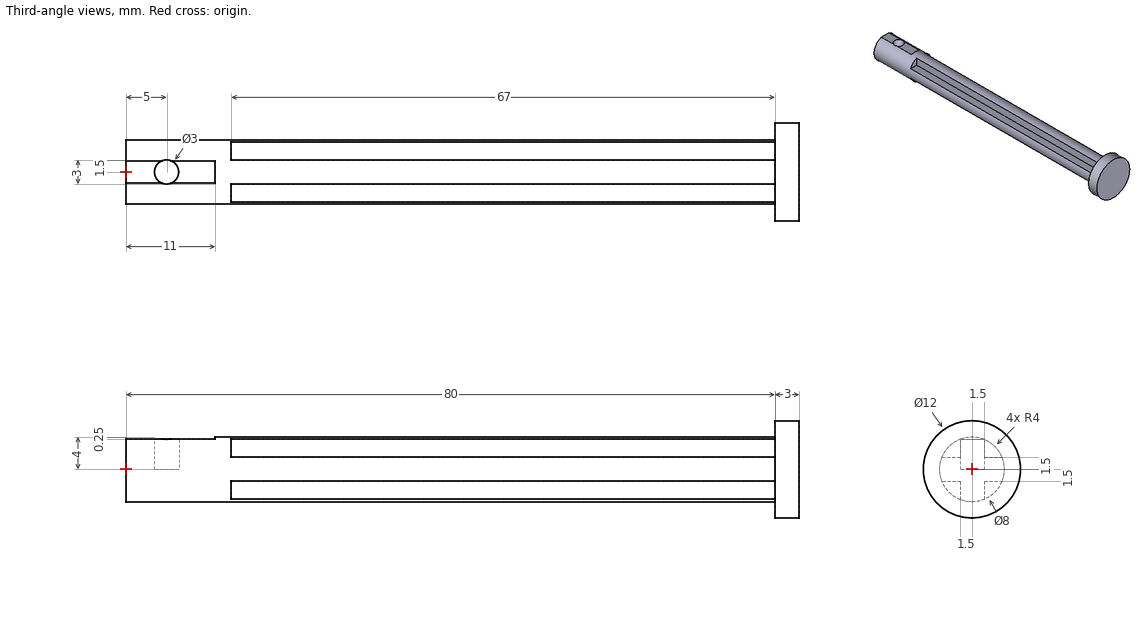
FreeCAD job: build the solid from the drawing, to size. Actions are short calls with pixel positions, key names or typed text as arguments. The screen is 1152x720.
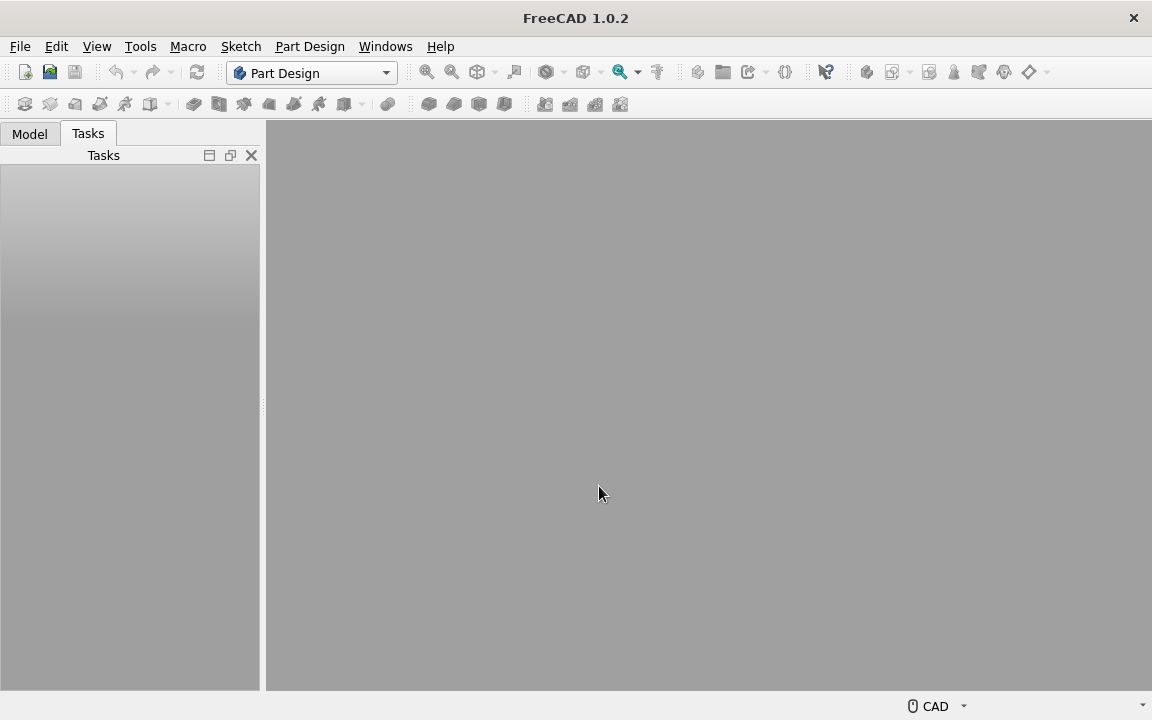
key(ctrl+n)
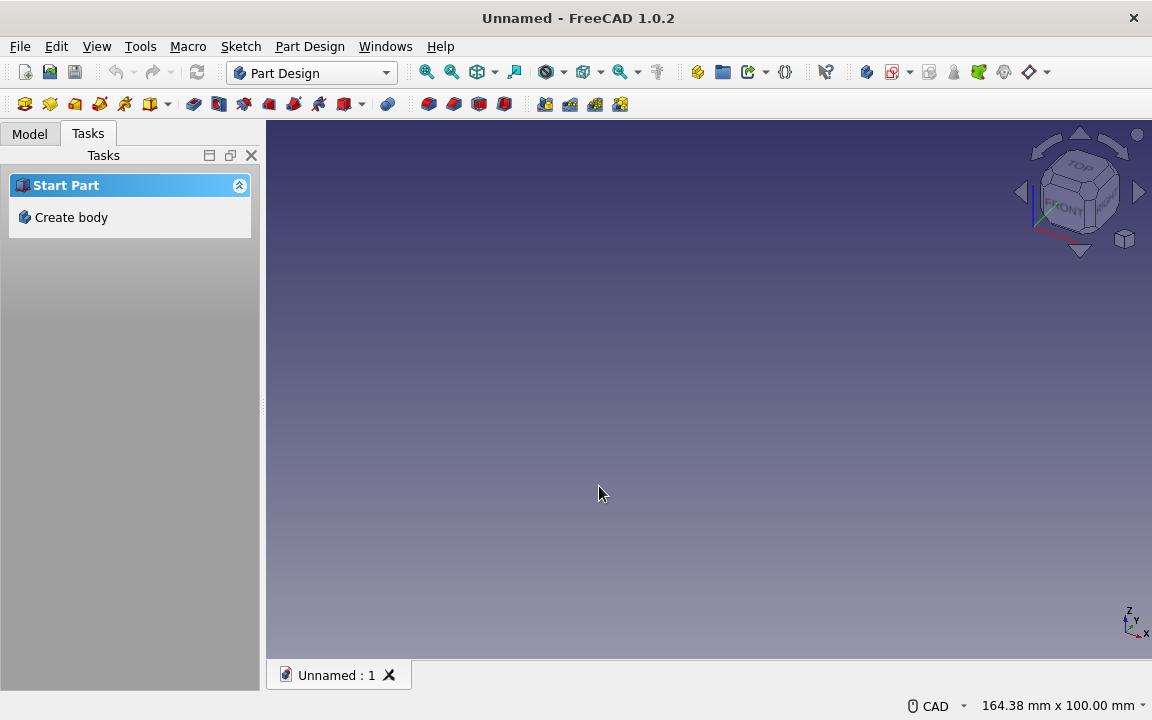
click(892, 72)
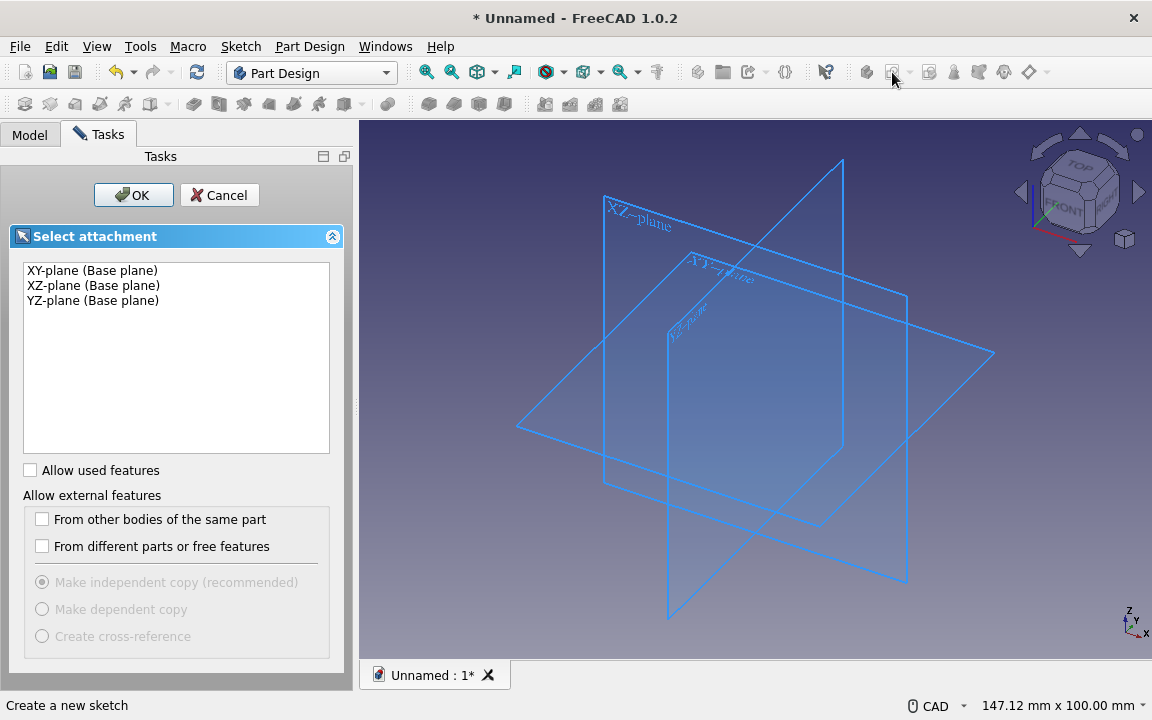
click(84, 300)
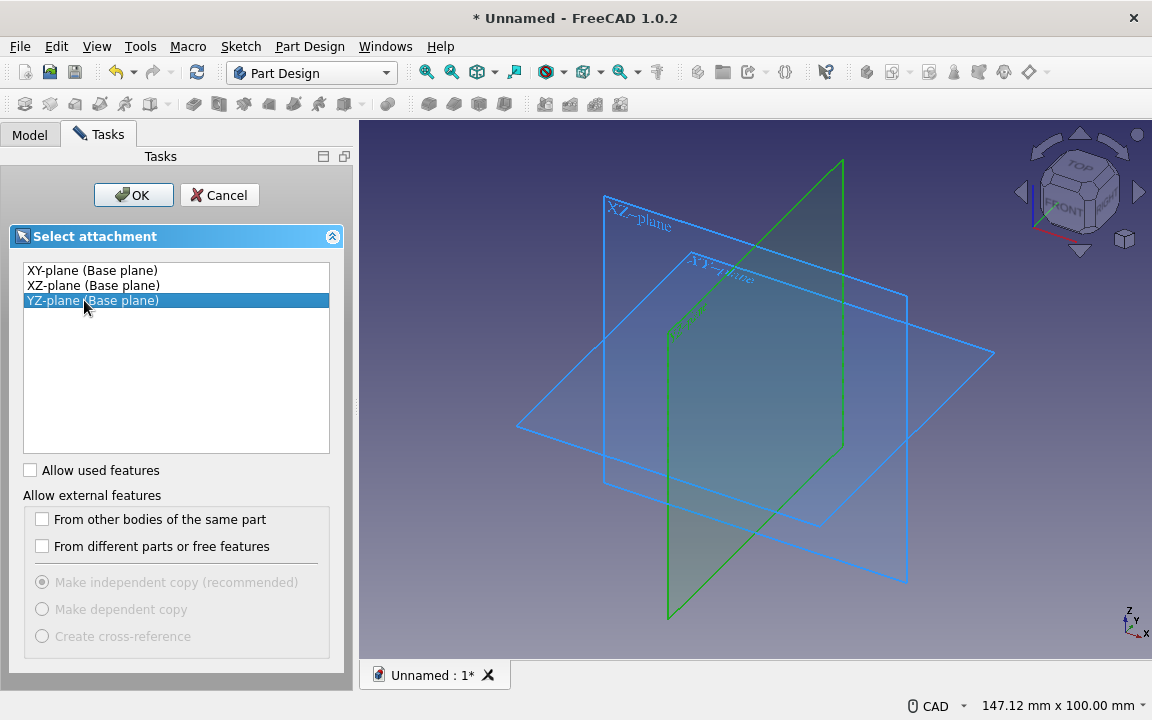
click(134, 195)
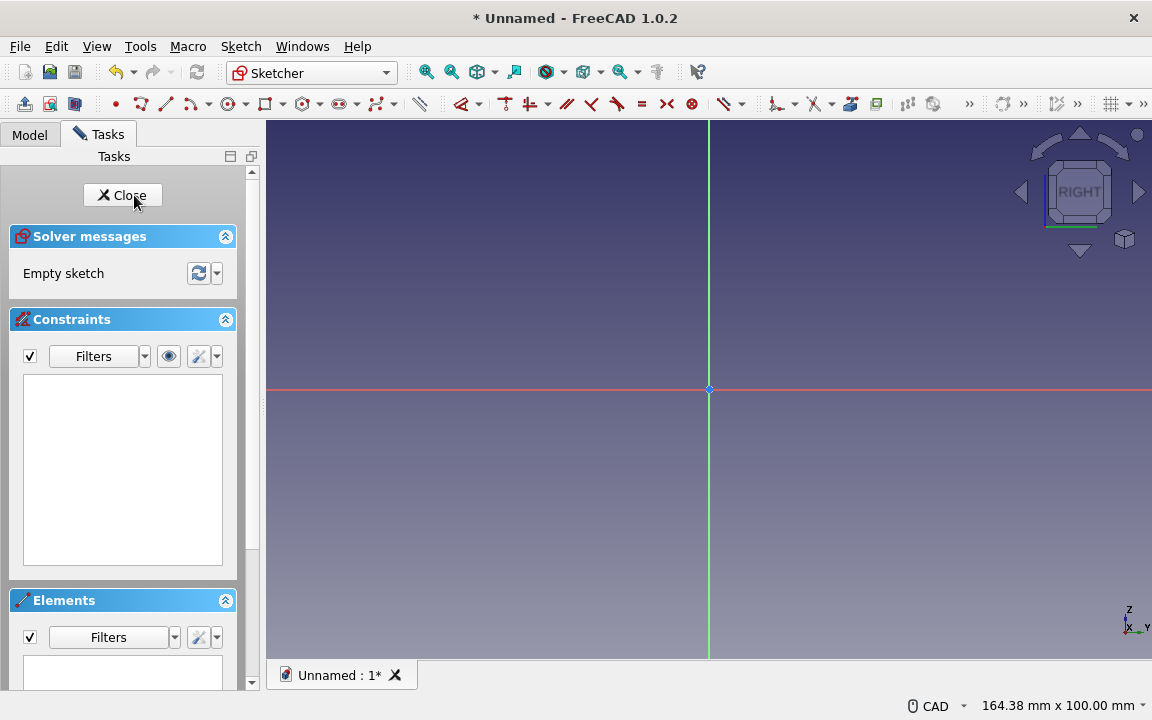
scroll(720, 390, up, 10)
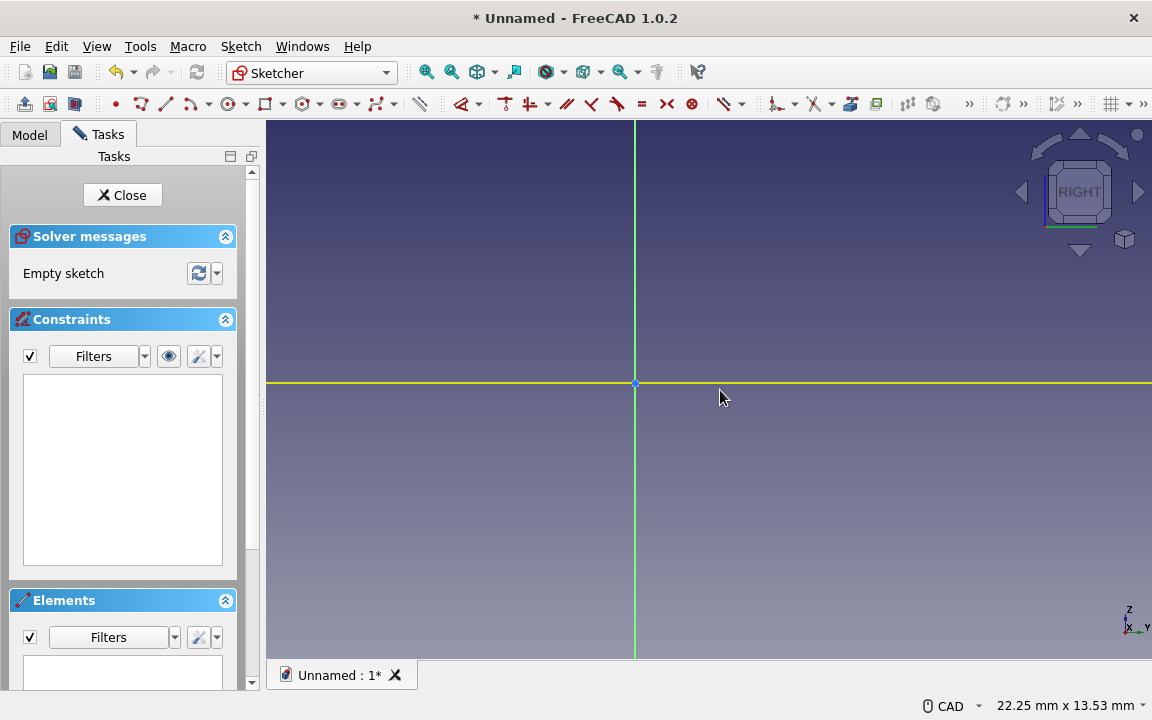
click(228, 104)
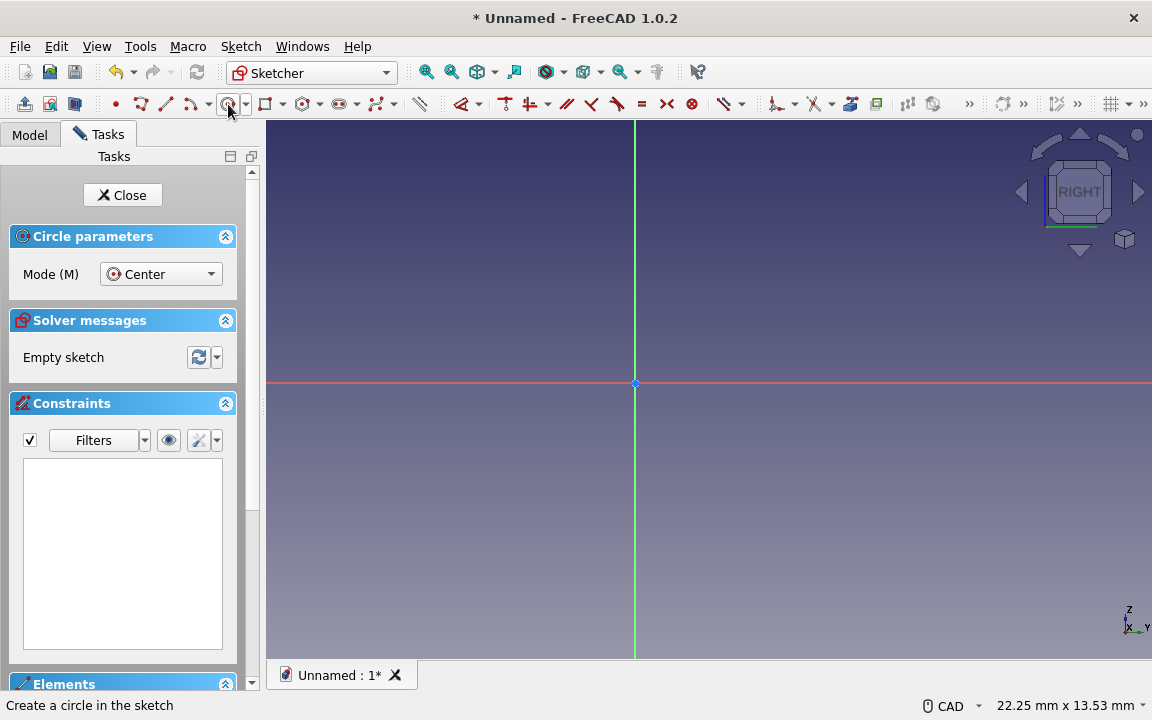
click(635, 383)
move(748, 270)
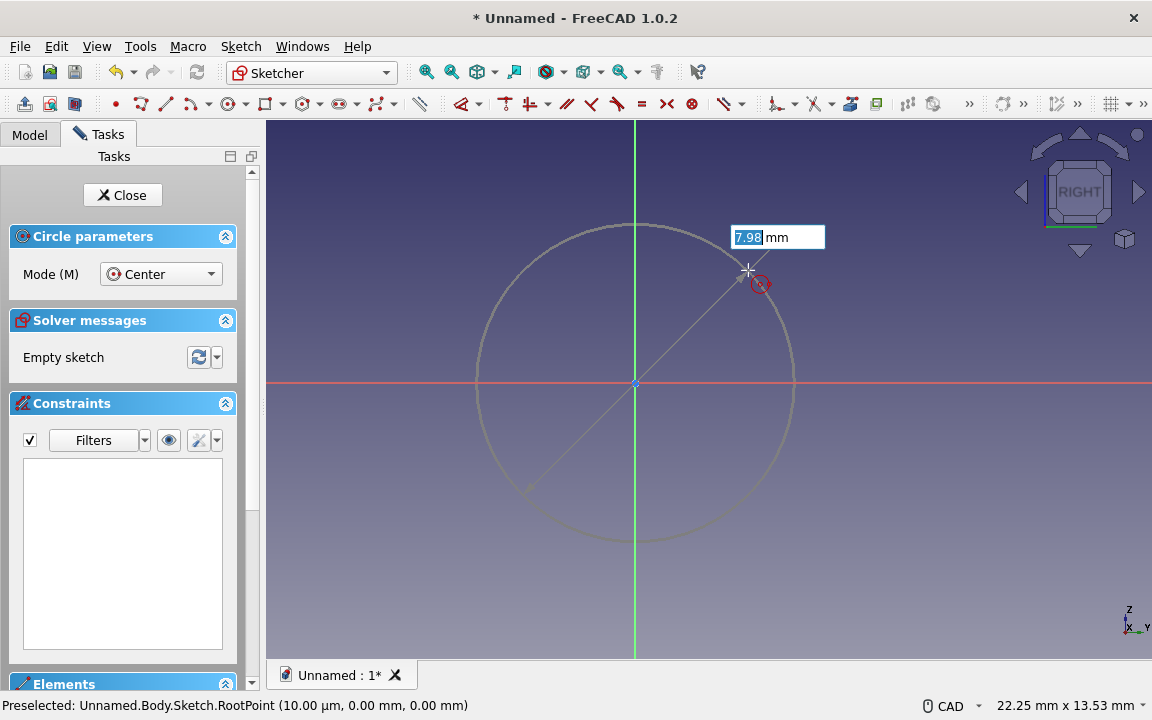
text(8)
key(Return)
key(Escape)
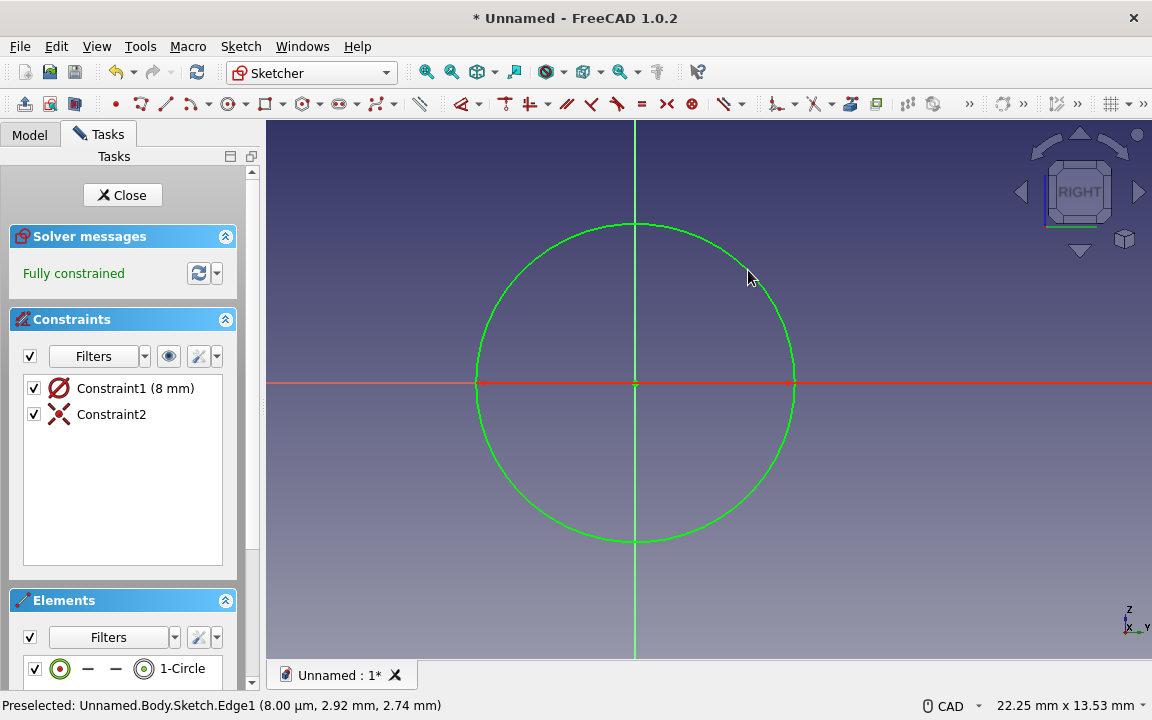
click(123, 195)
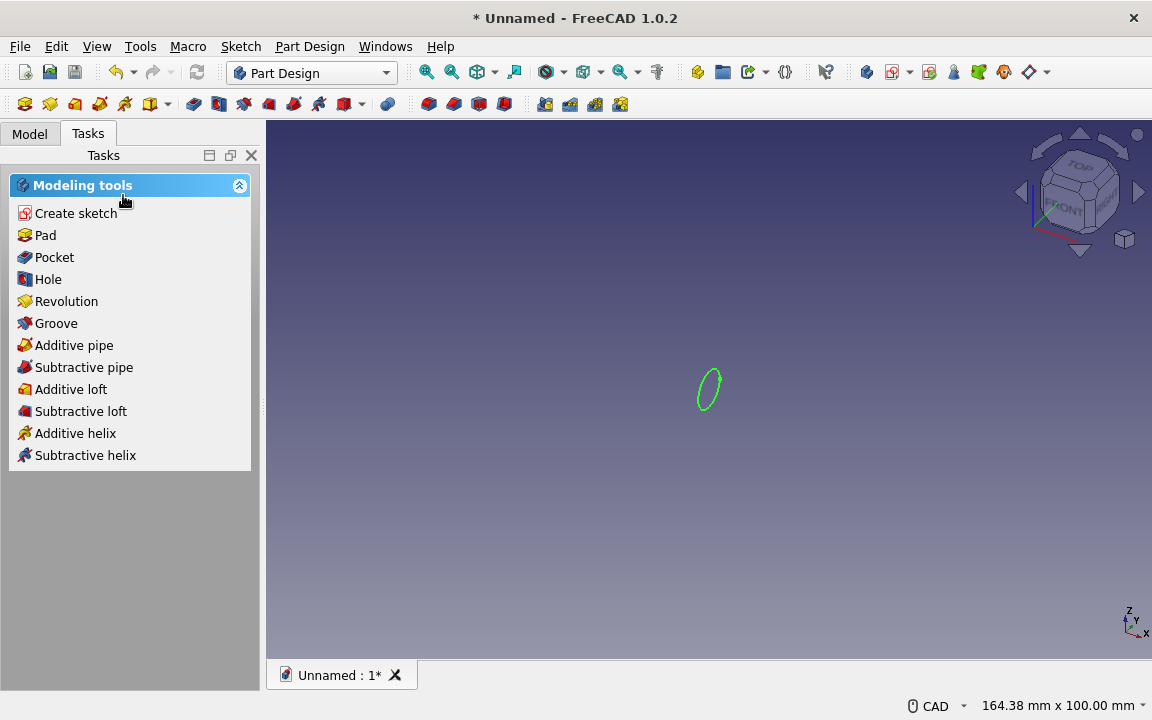
click(25, 104)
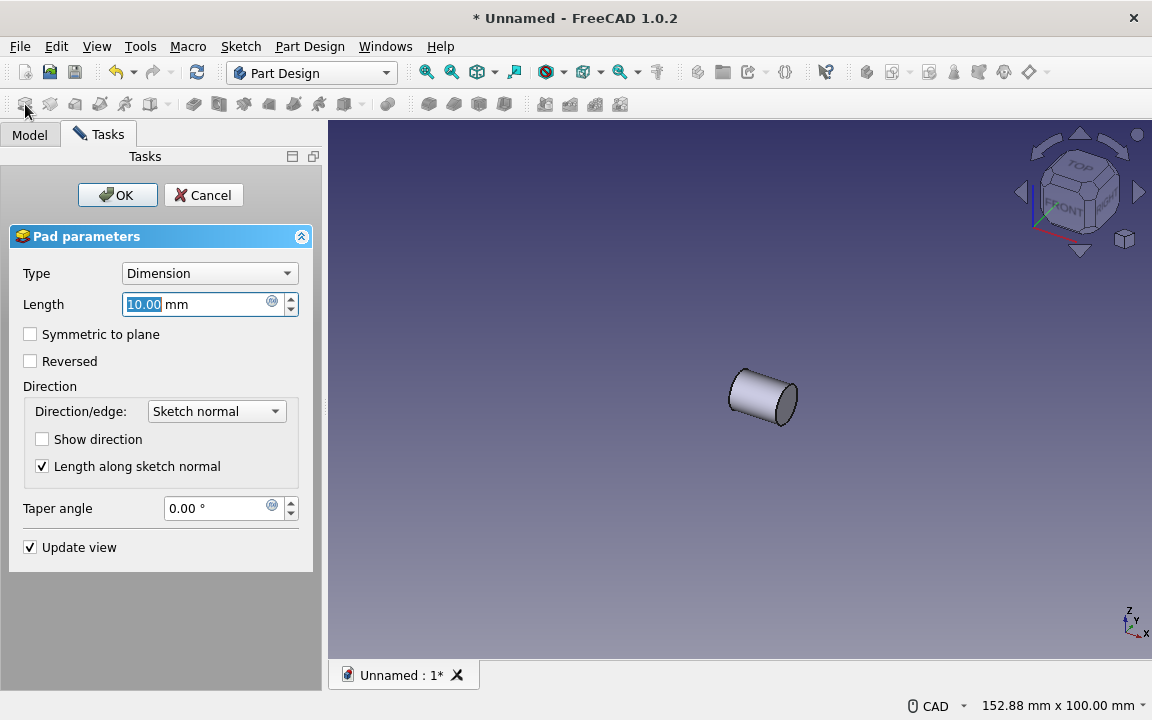
text(80)
key(Tab)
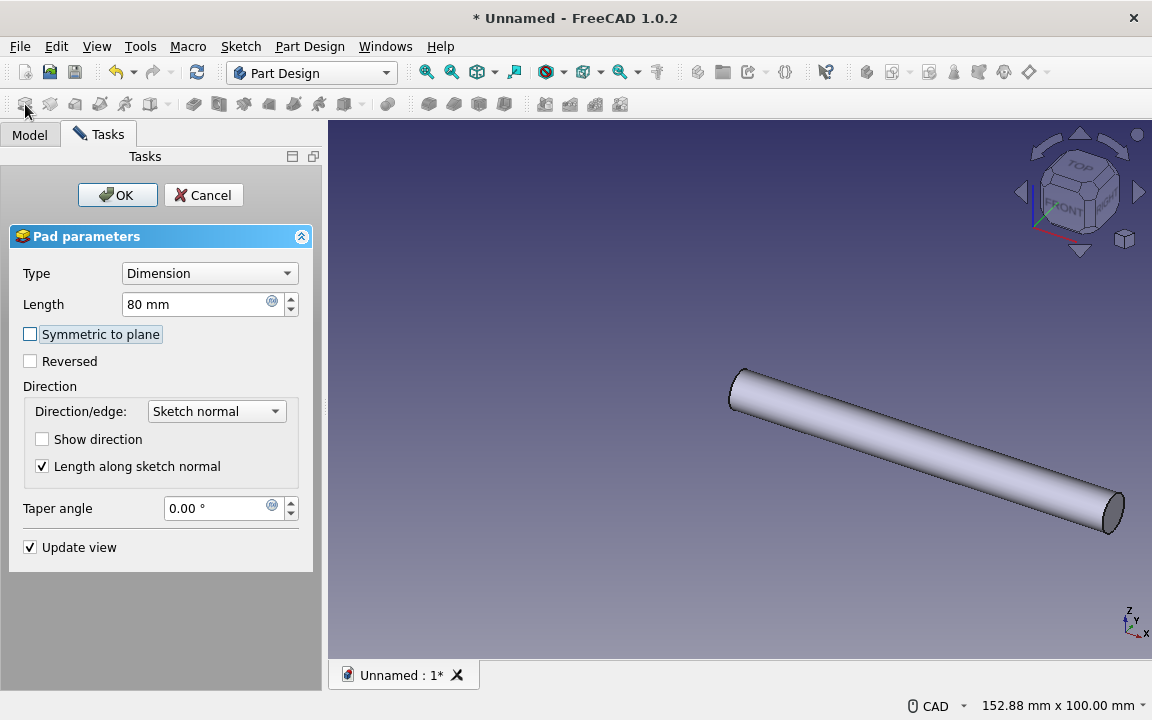
click(118, 195)